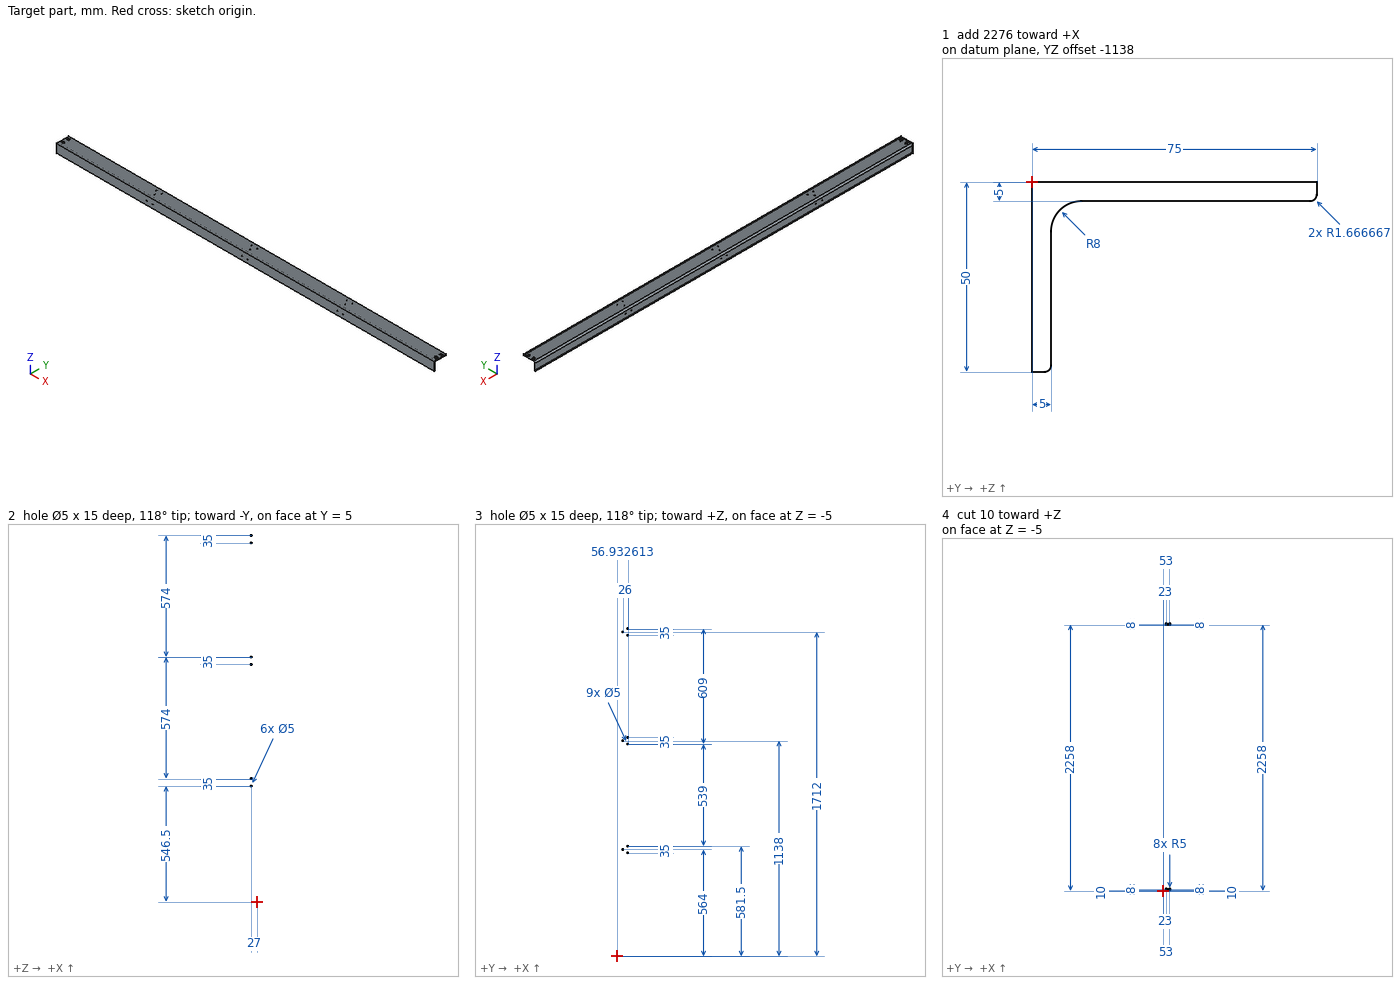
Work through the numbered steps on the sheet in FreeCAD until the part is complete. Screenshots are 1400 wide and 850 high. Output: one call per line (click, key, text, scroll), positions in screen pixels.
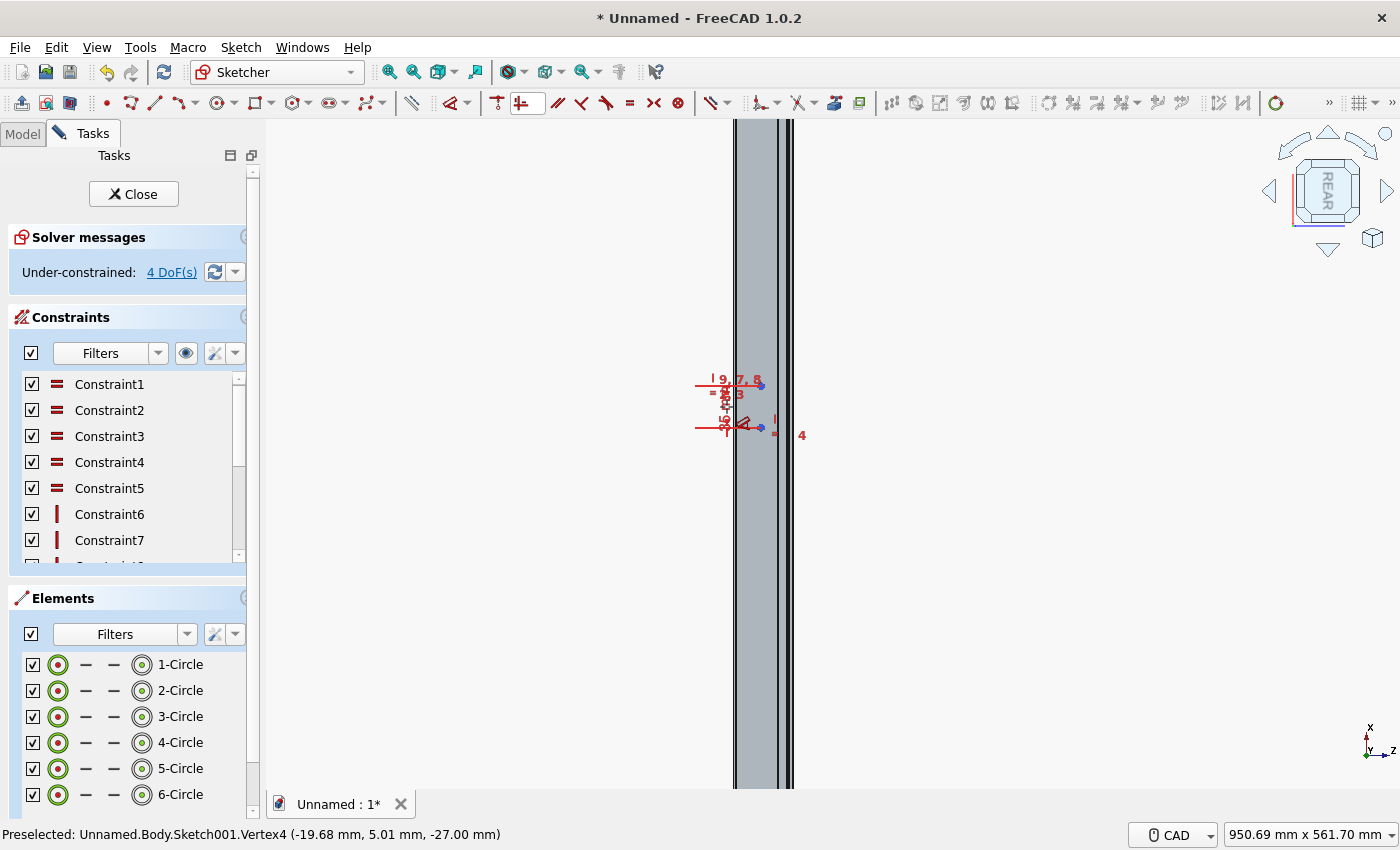
scroll(762, 384, down, 8)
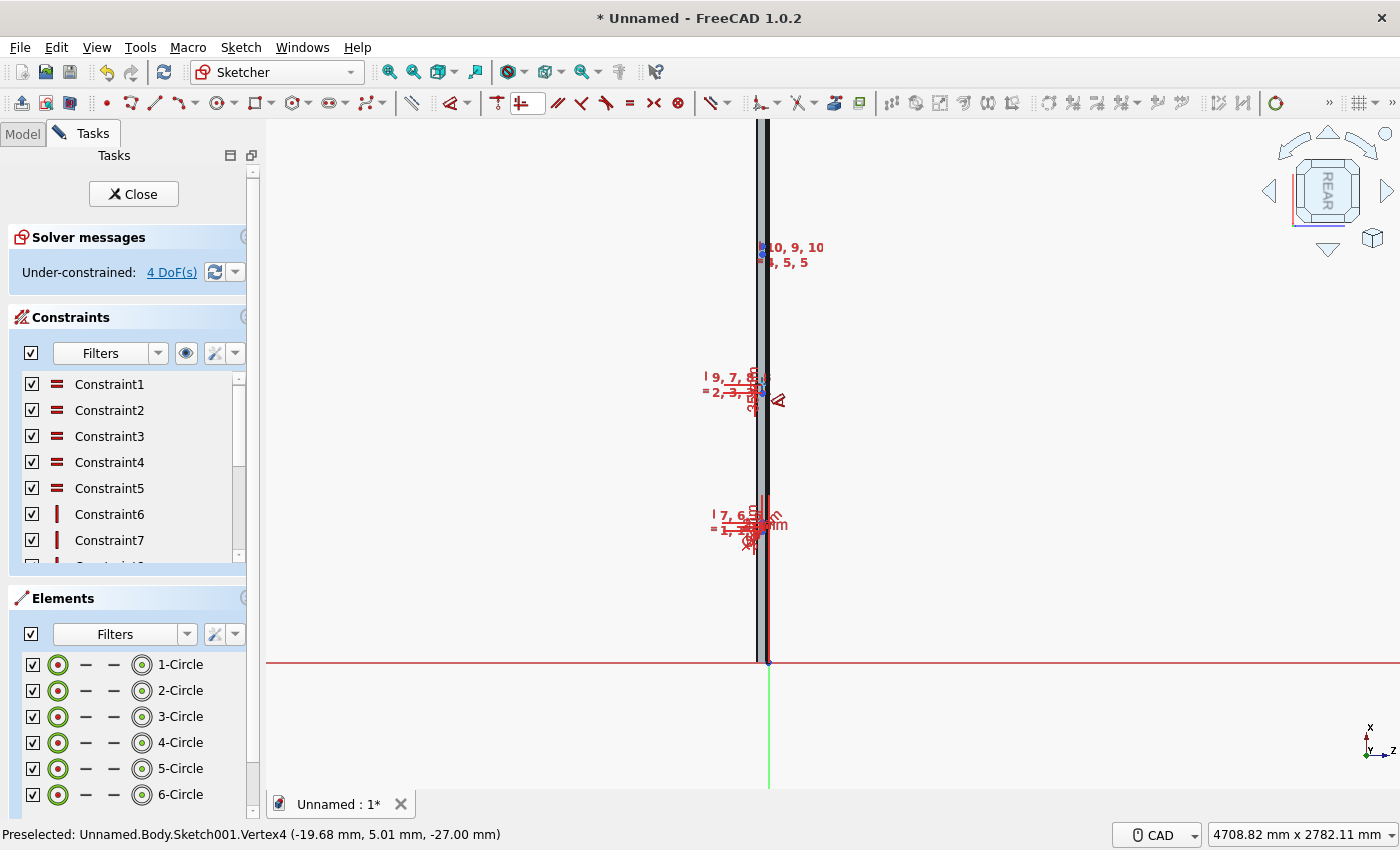
scroll(762, 246, up, 8)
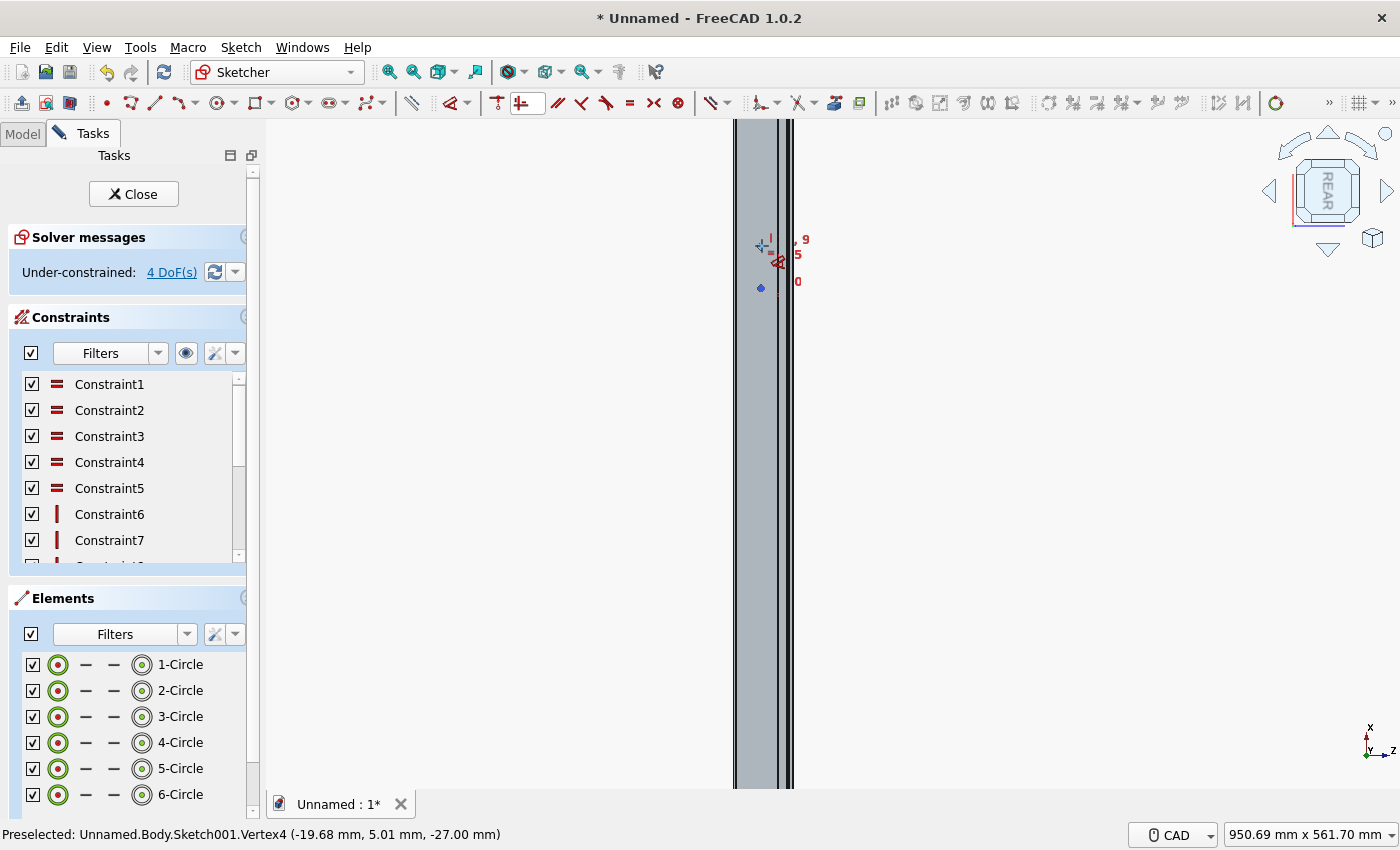
click(761, 247)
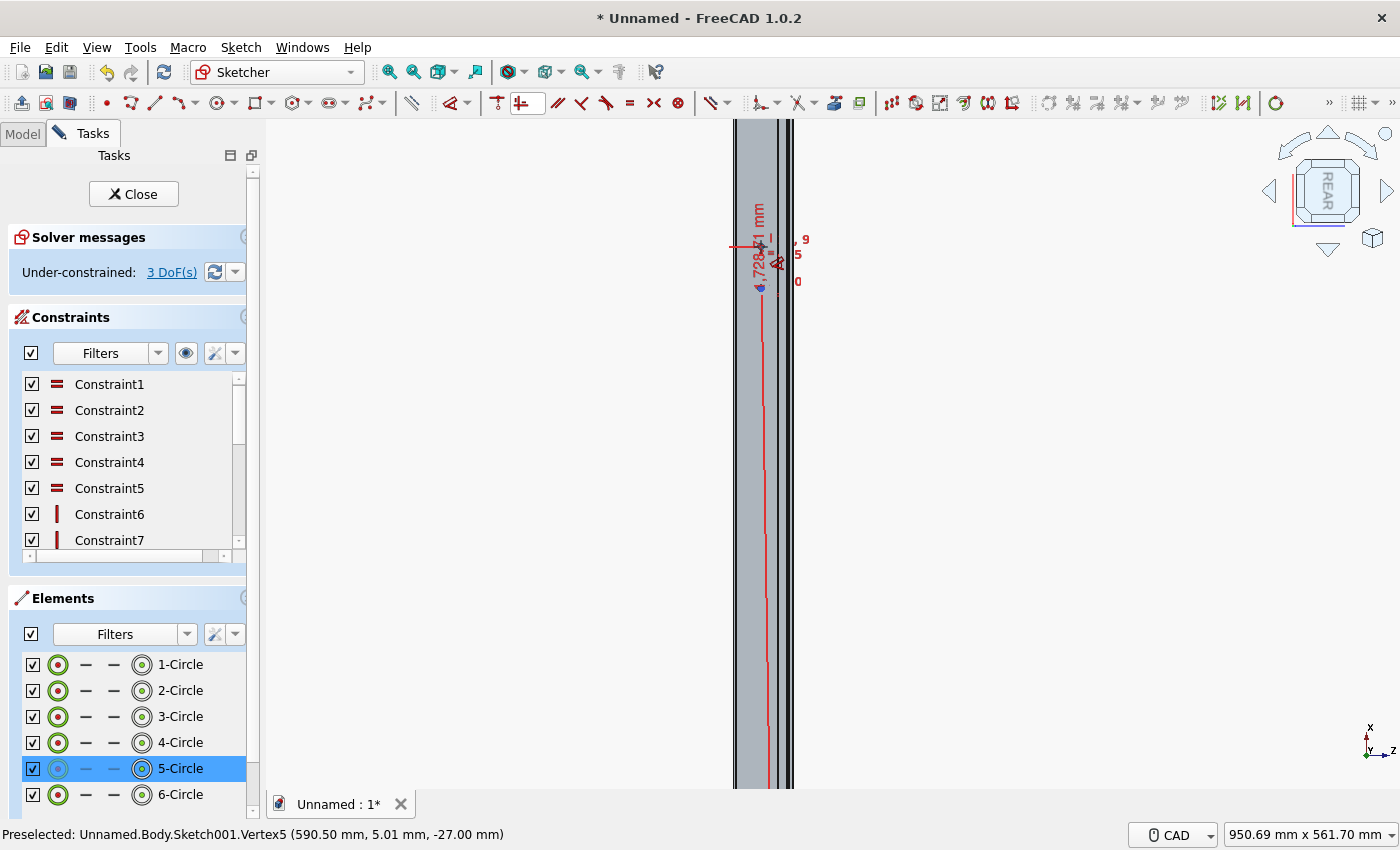
click(761, 288)
click(727, 268)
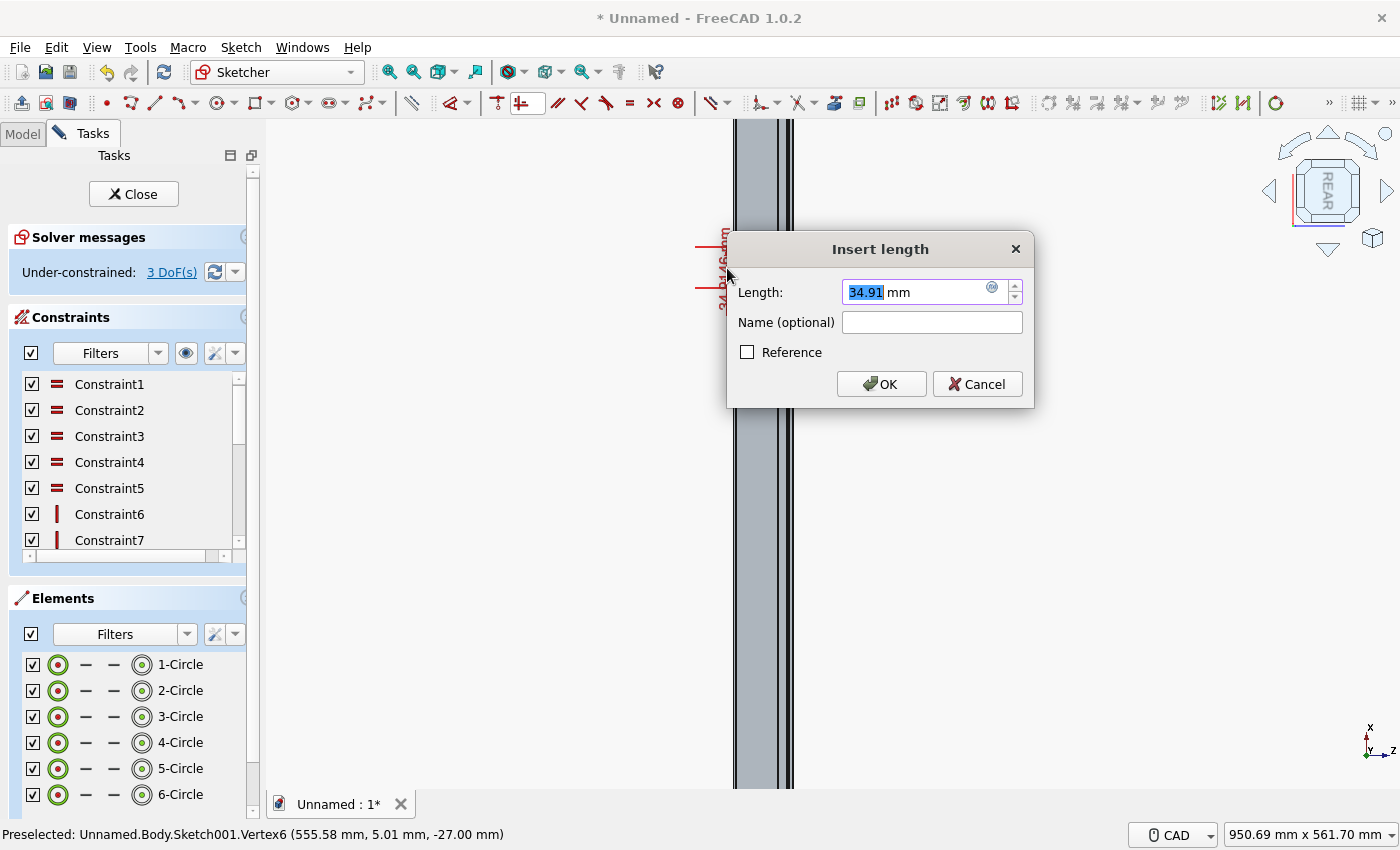
text(35)
key(Return)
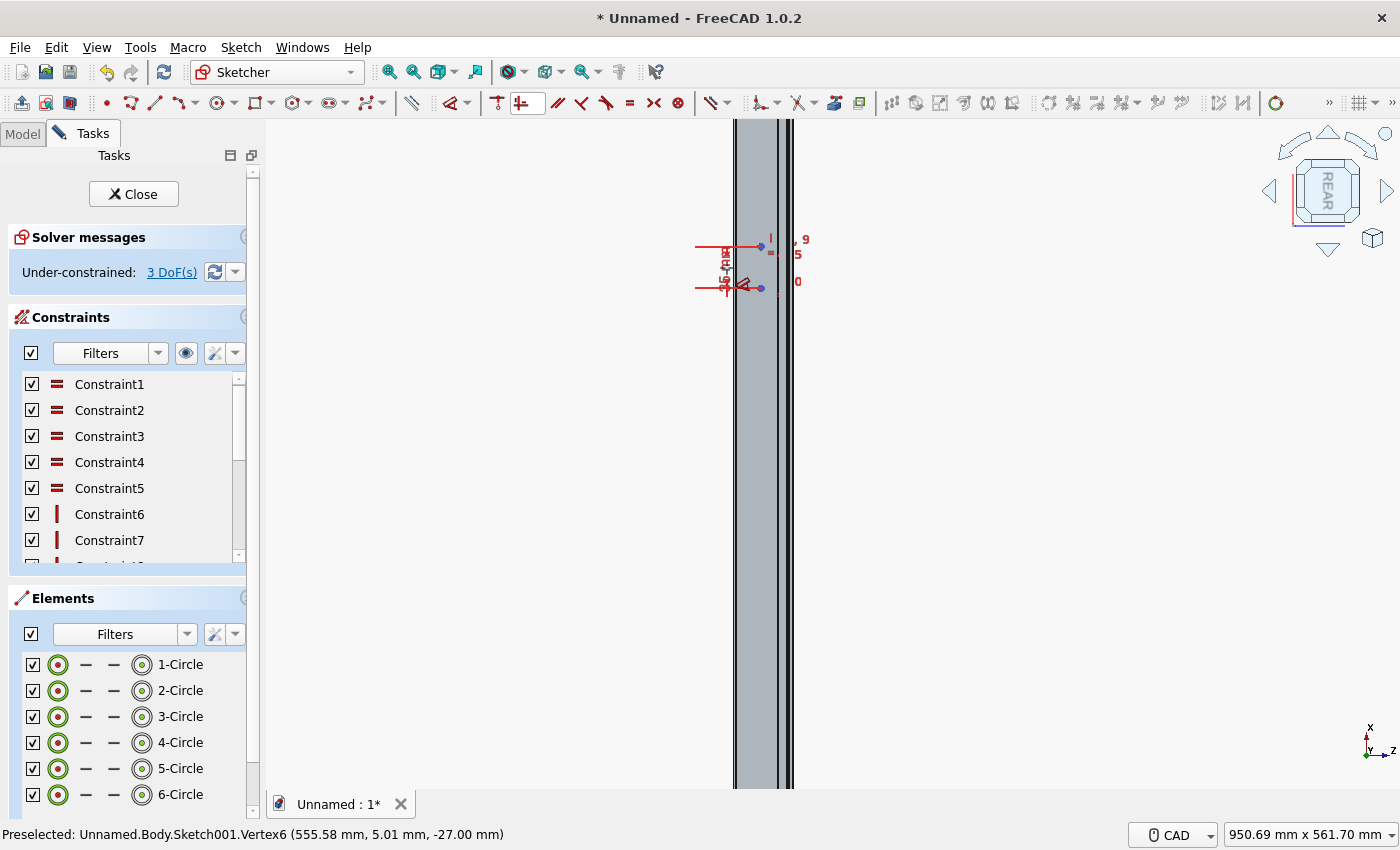
scroll(762, 246, down, 8)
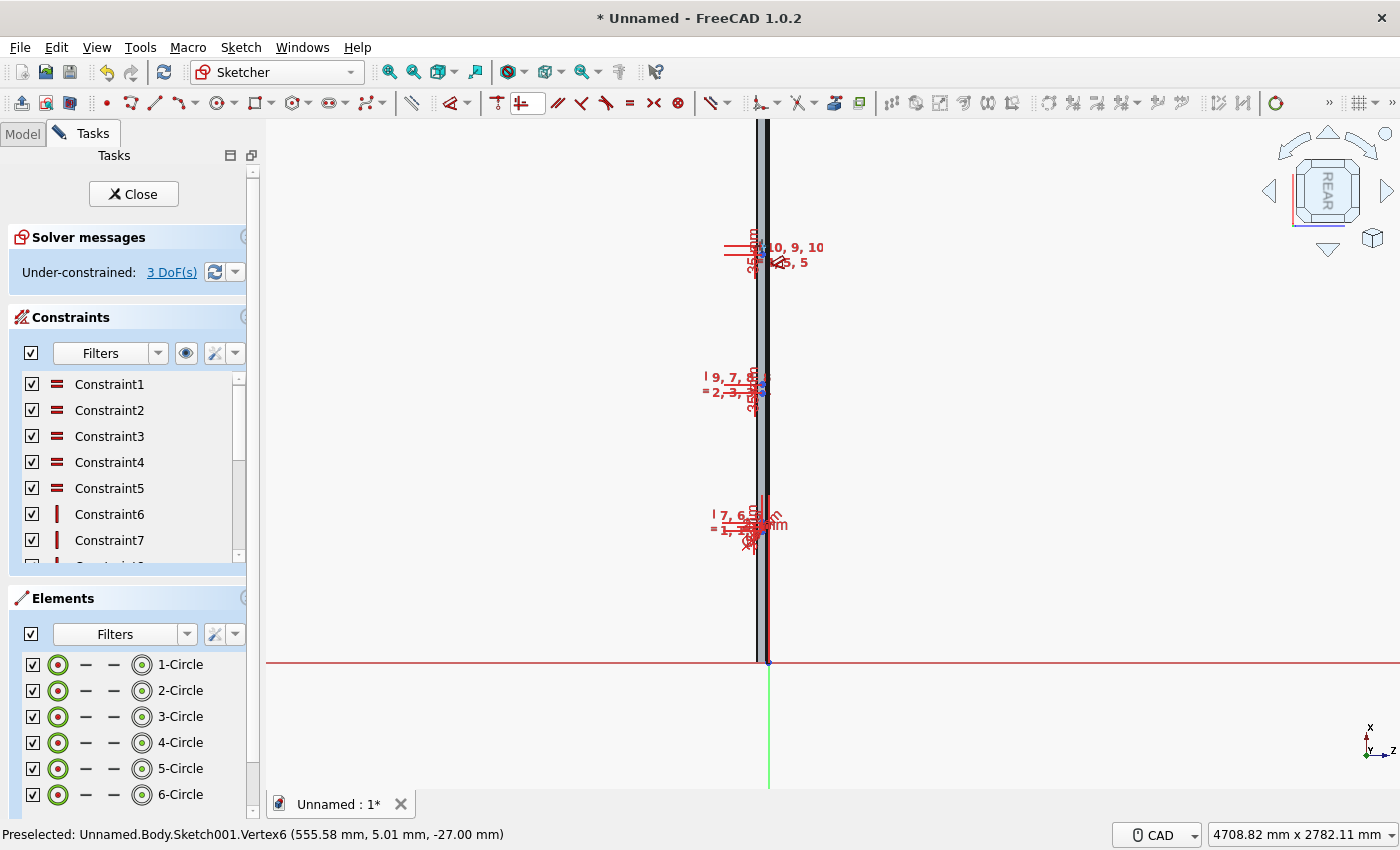
scroll(762, 523, up, 2)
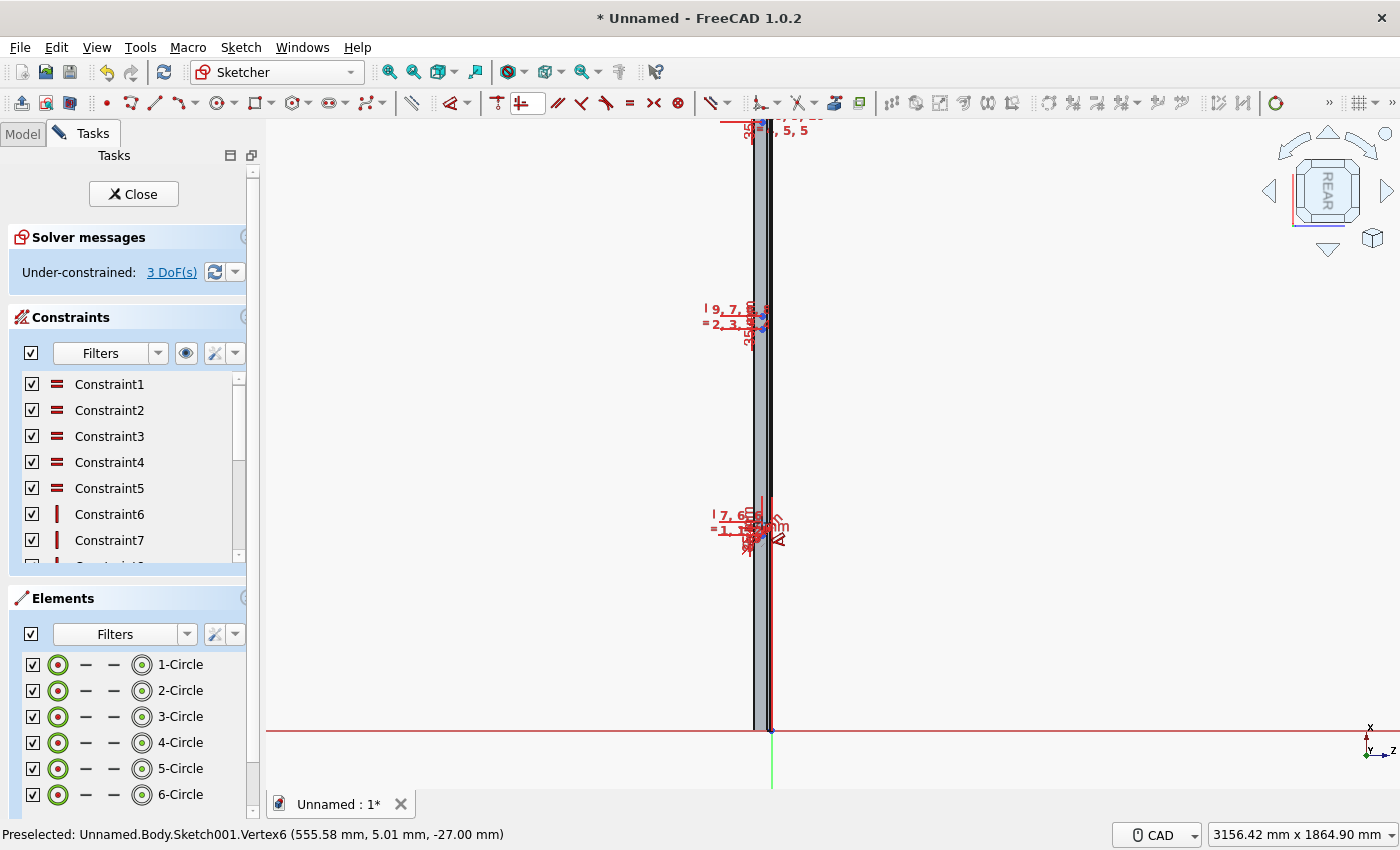
click(762, 522)